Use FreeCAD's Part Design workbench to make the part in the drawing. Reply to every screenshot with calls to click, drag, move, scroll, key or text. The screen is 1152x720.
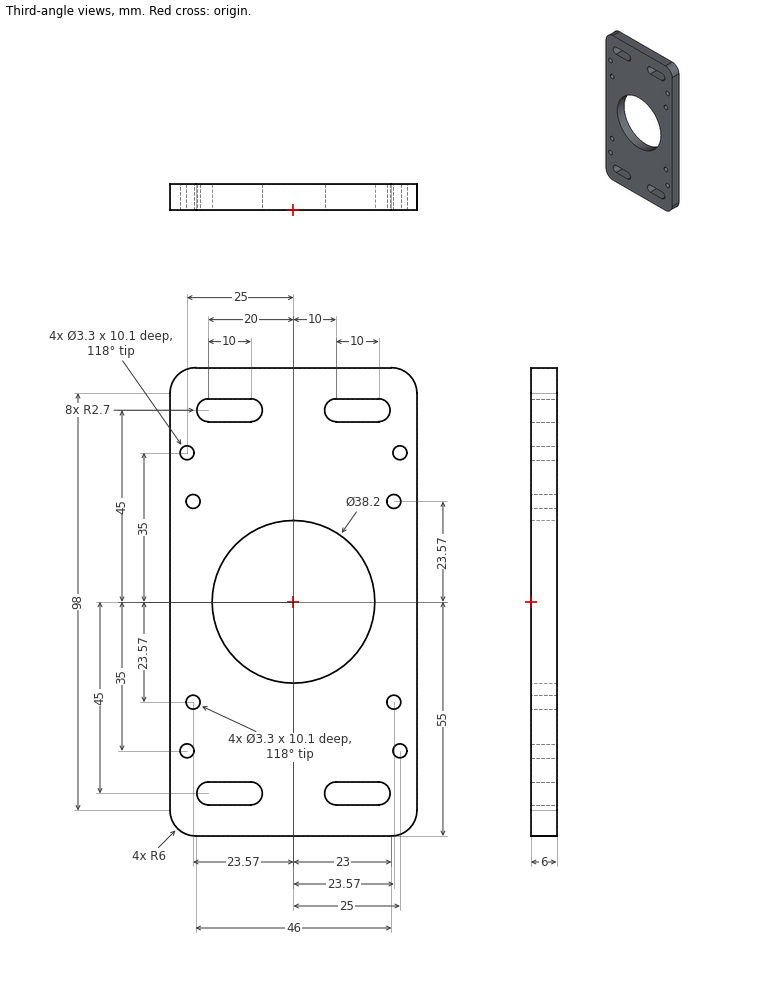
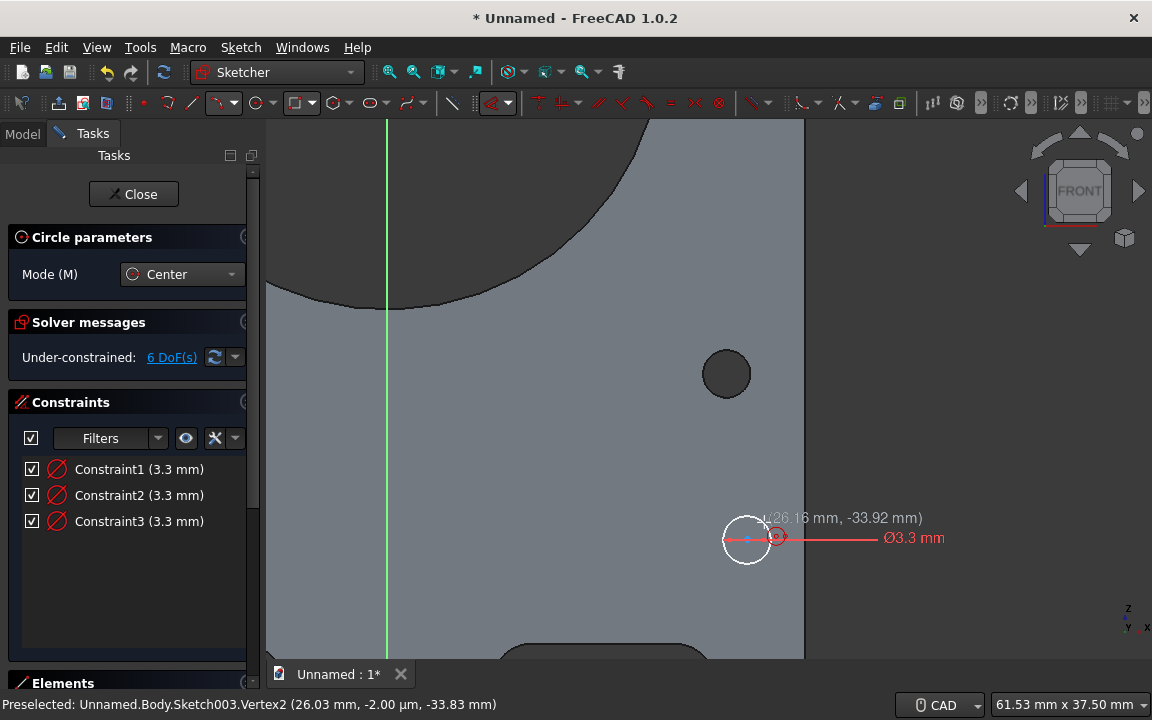
scroll(750, 542, down, 6)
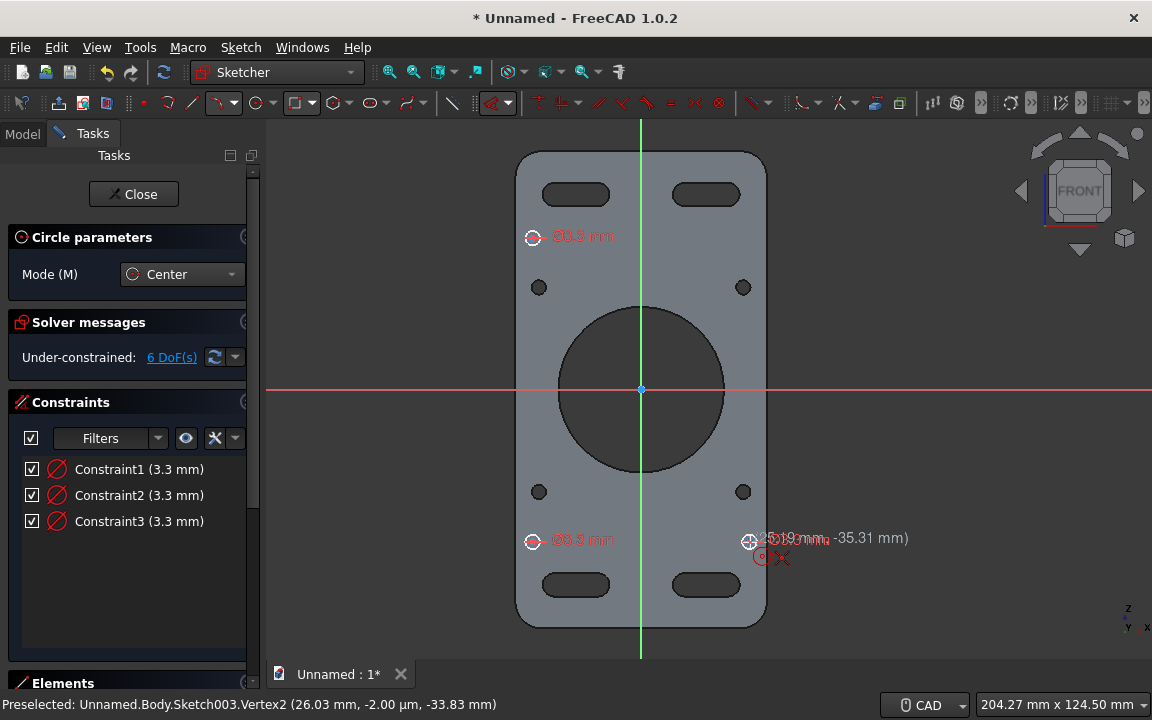
scroll(750, 238, up, 6)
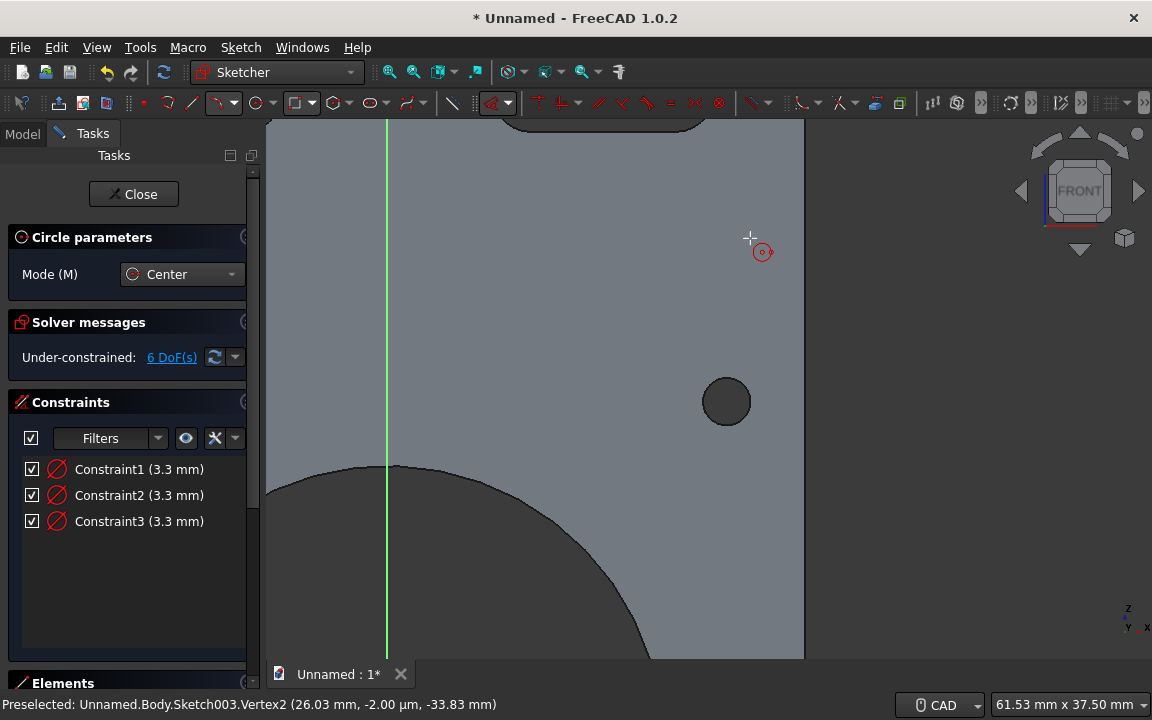
click(747, 237)
move(764, 220)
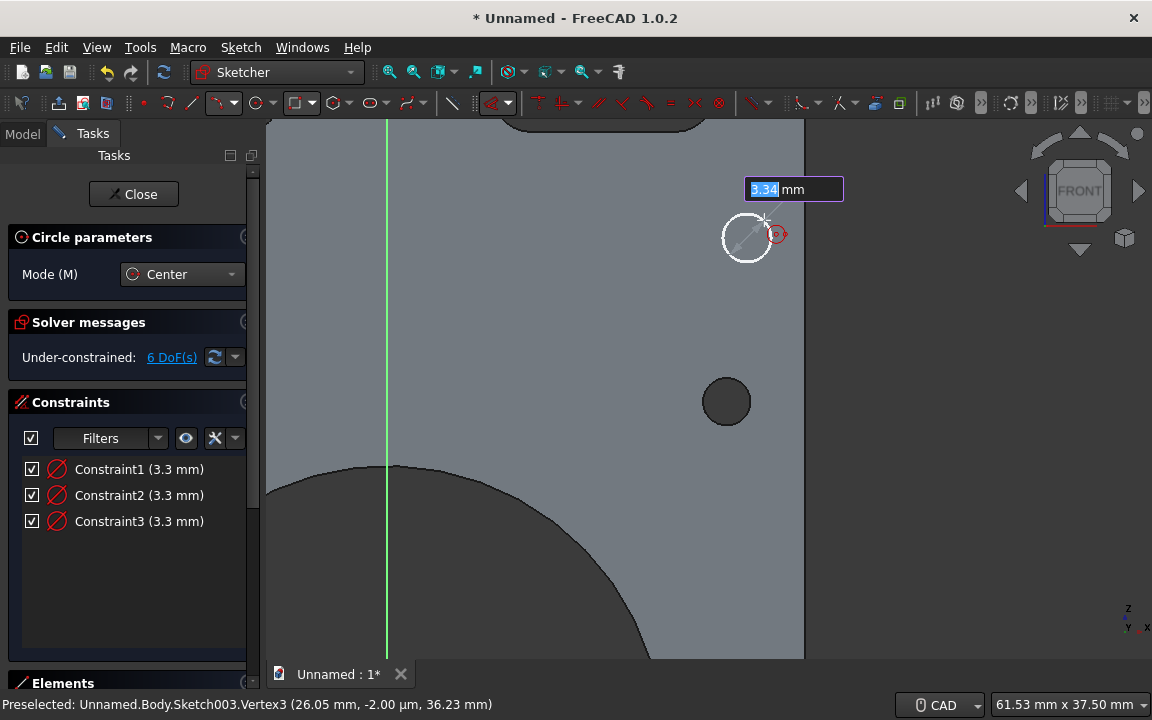
text(3.3)
key(Return)
key(Escape)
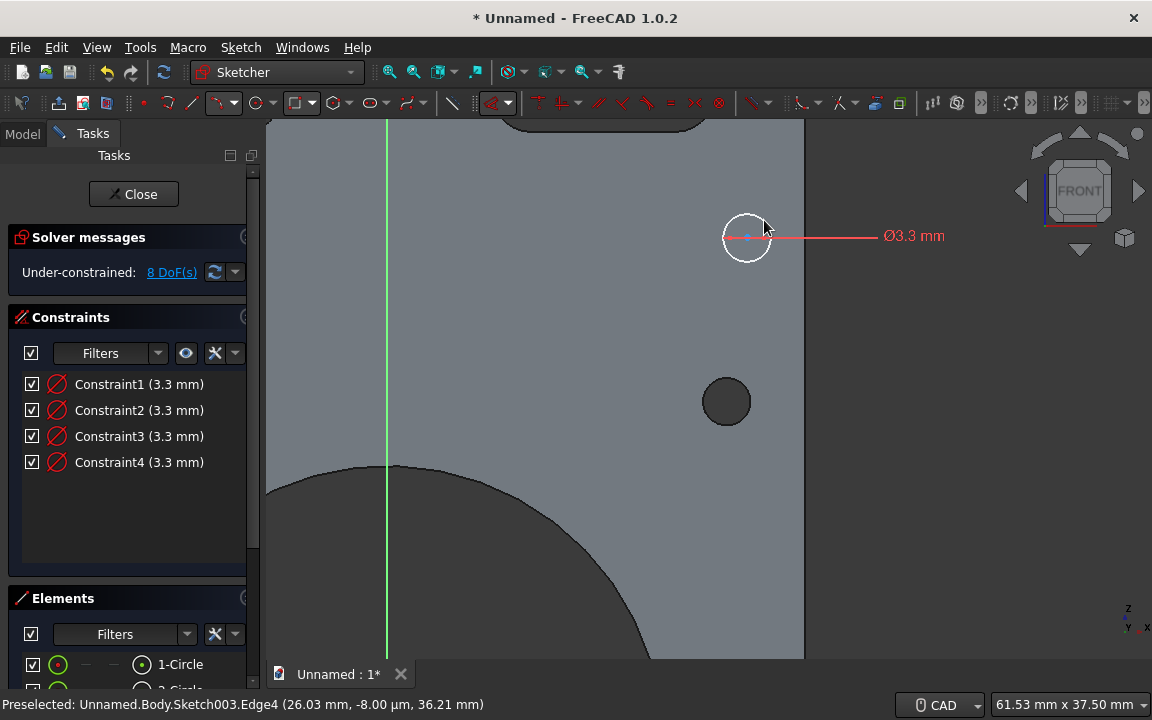
scroll(750, 237, down, 6)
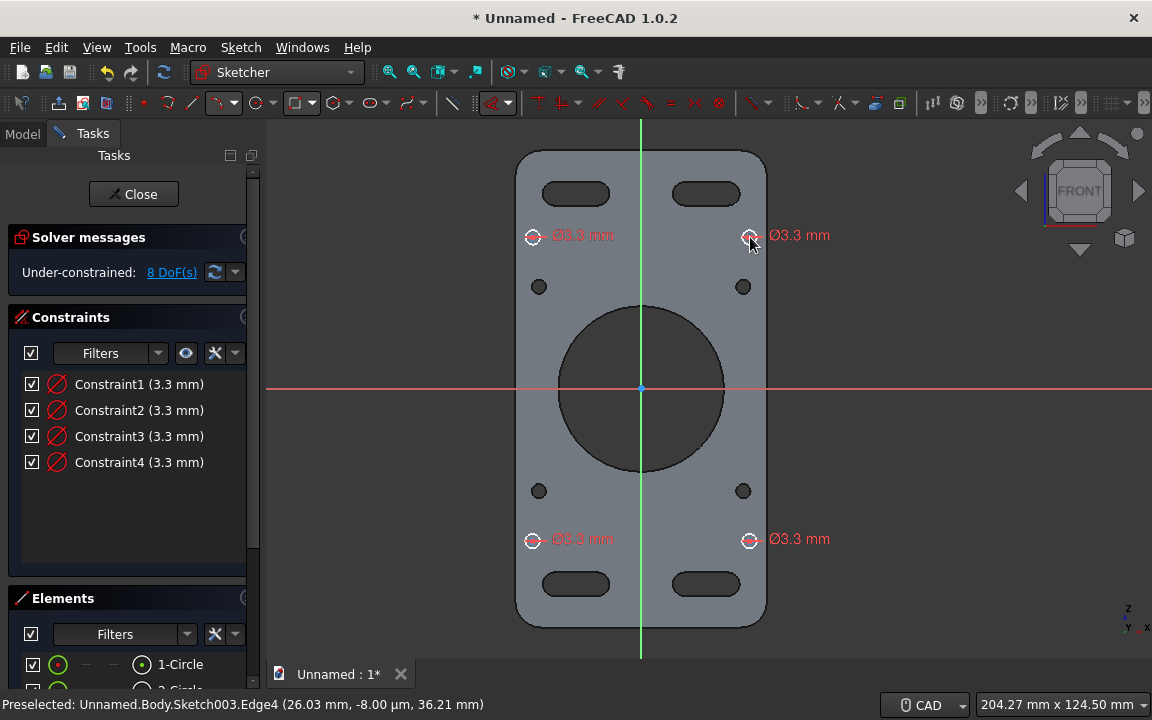
click(533, 237)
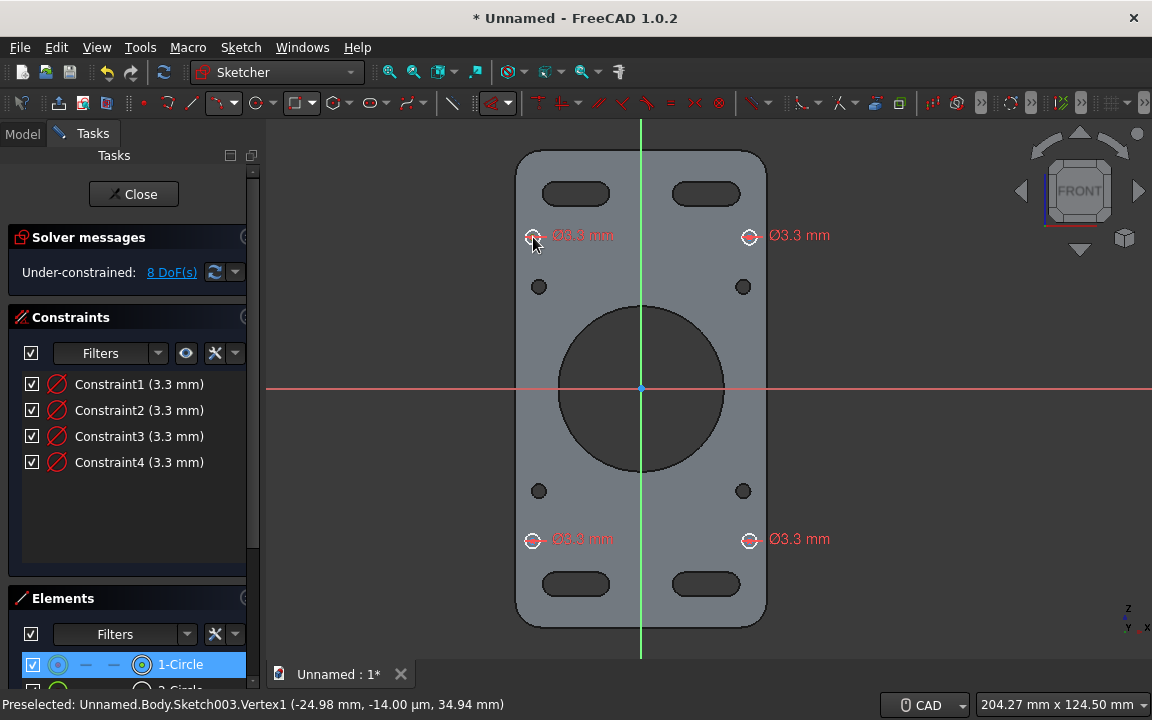
key(l)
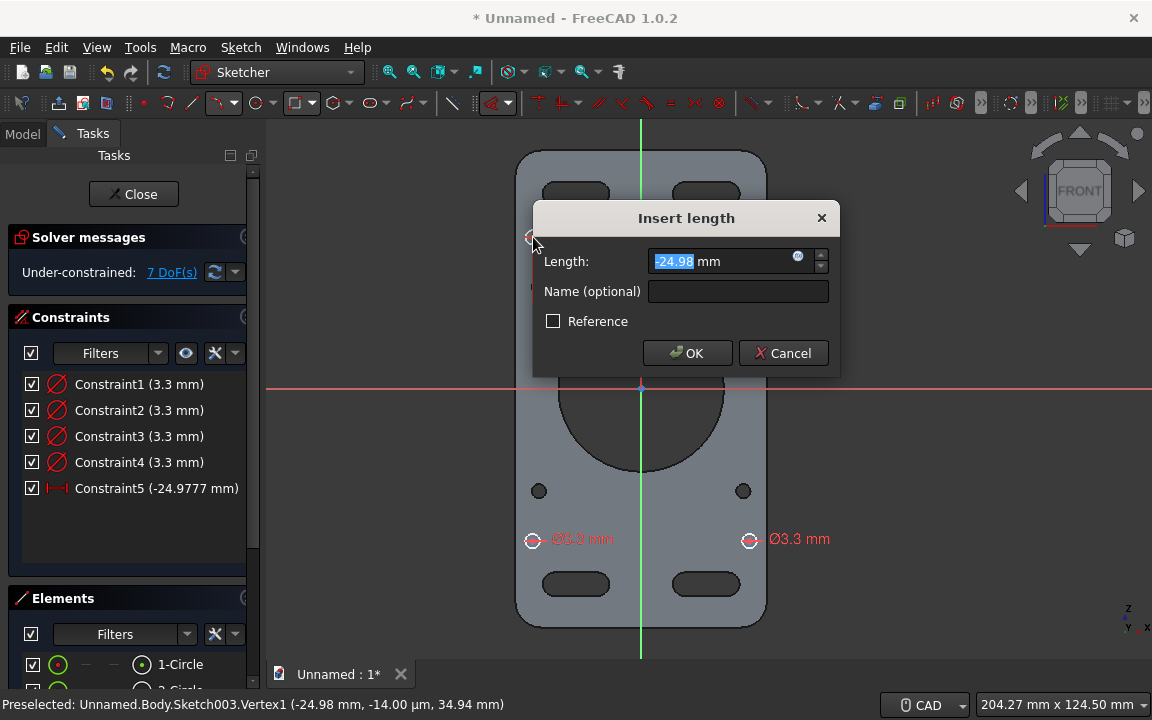
text(-25)
key(Return)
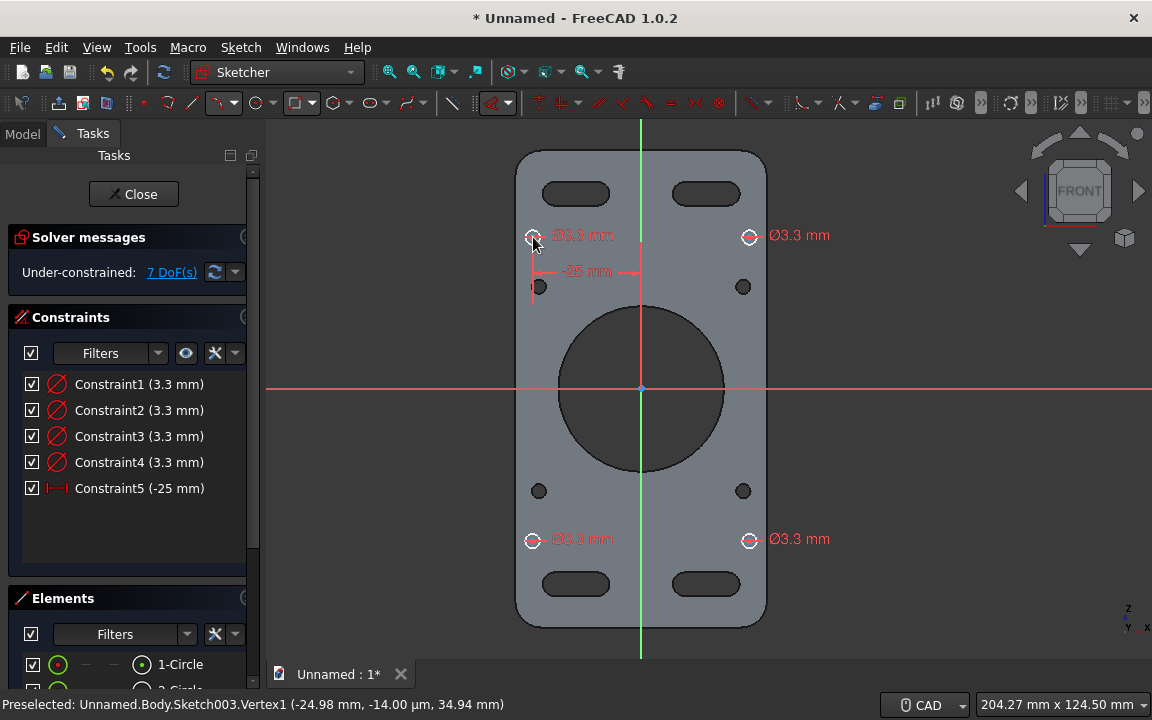
click(533, 237)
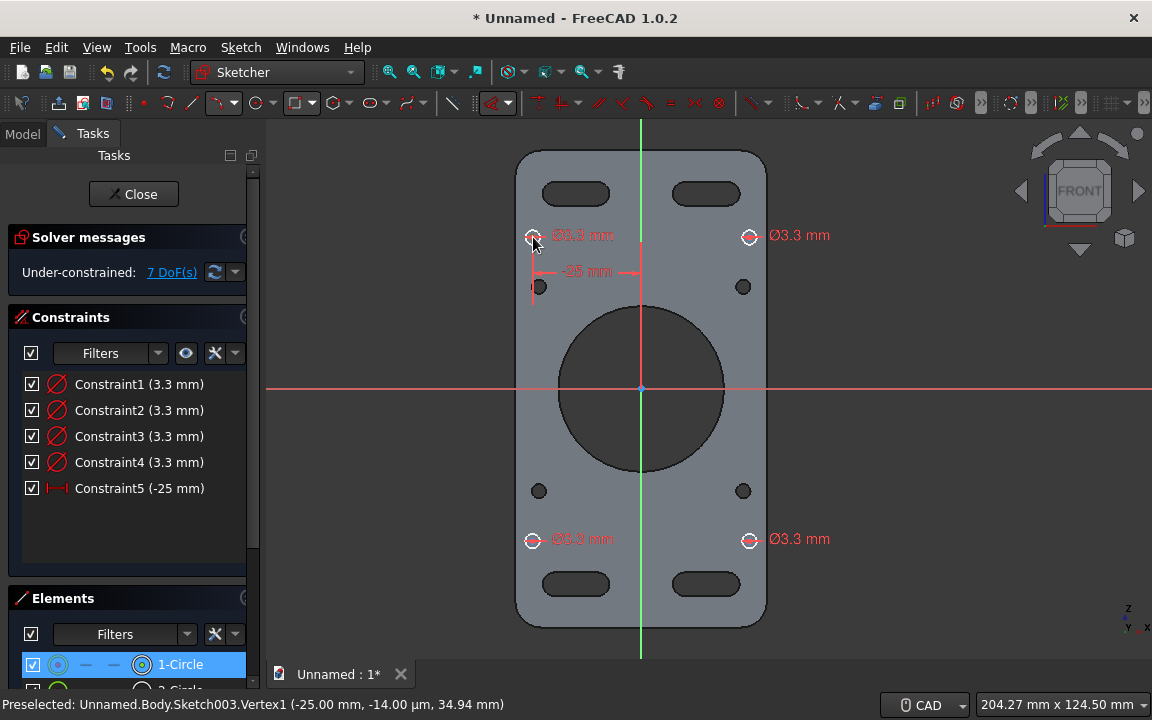
key(i)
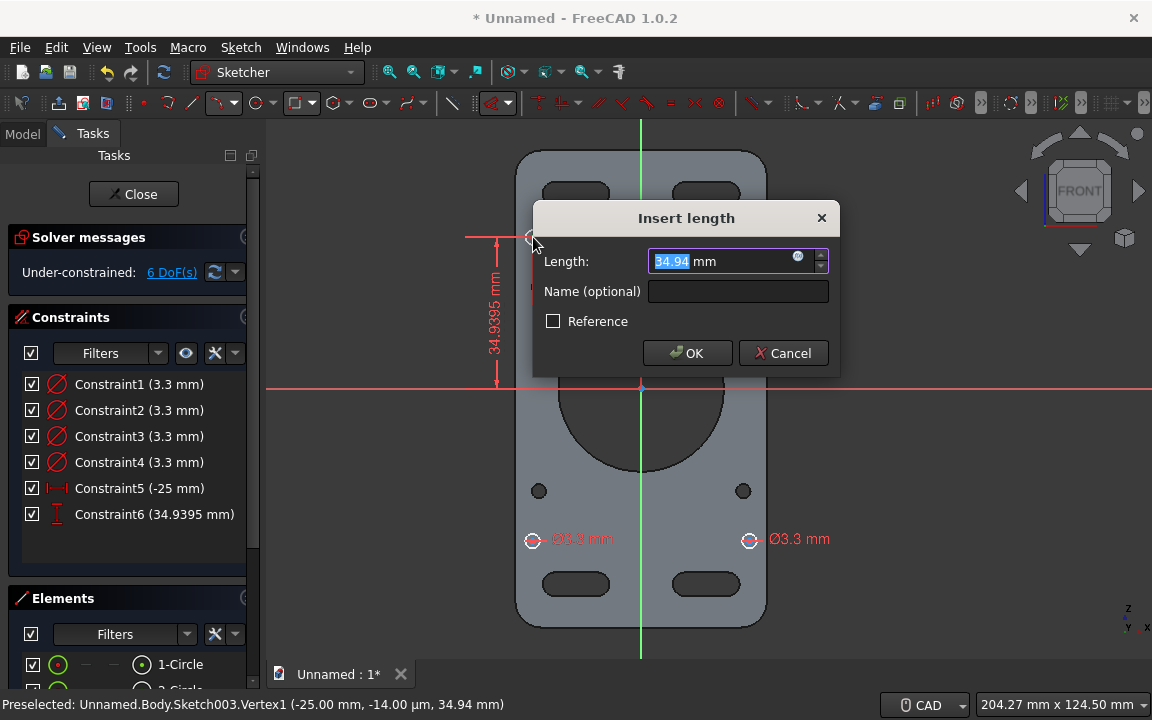
text(35)
key(Return)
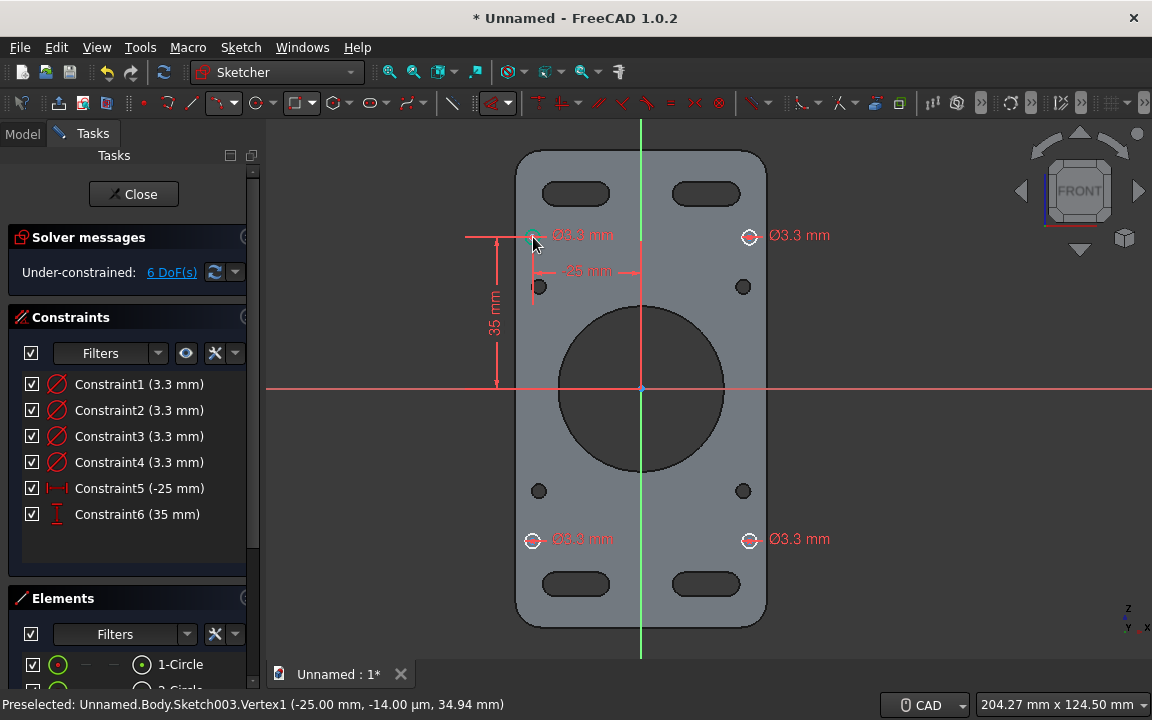
click(533, 541)